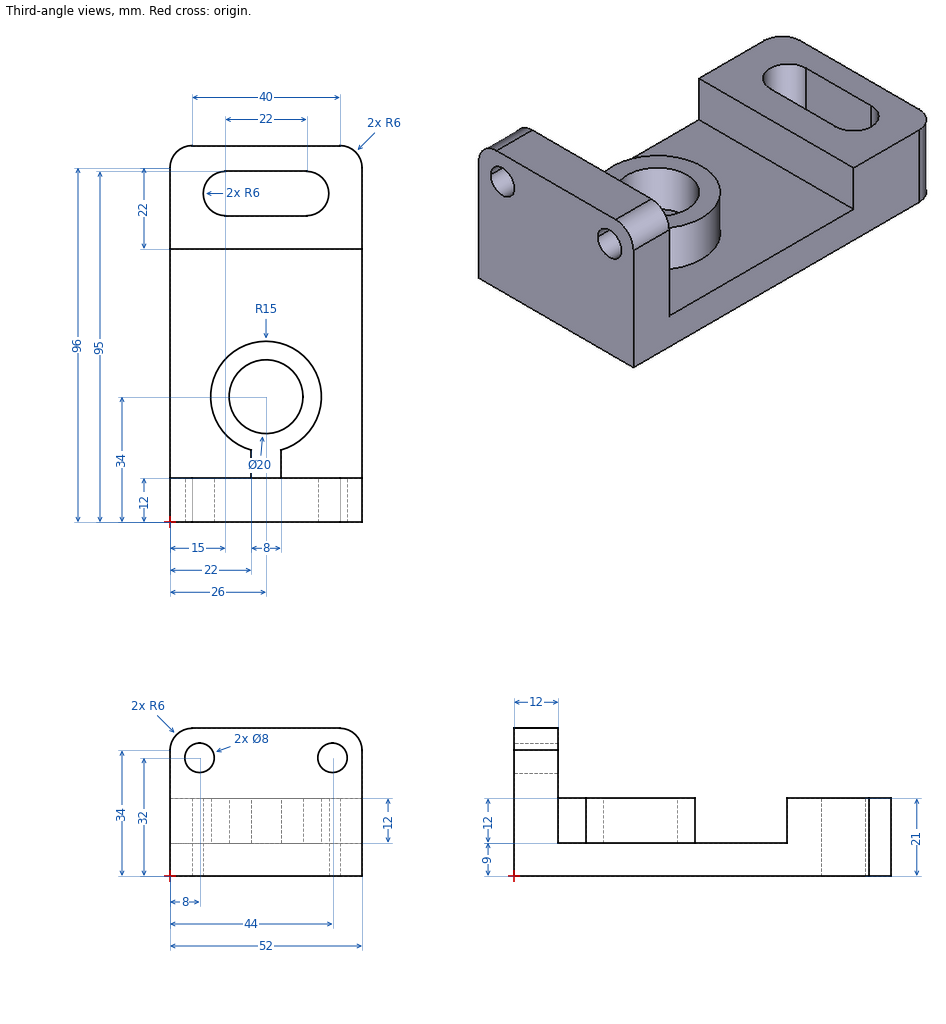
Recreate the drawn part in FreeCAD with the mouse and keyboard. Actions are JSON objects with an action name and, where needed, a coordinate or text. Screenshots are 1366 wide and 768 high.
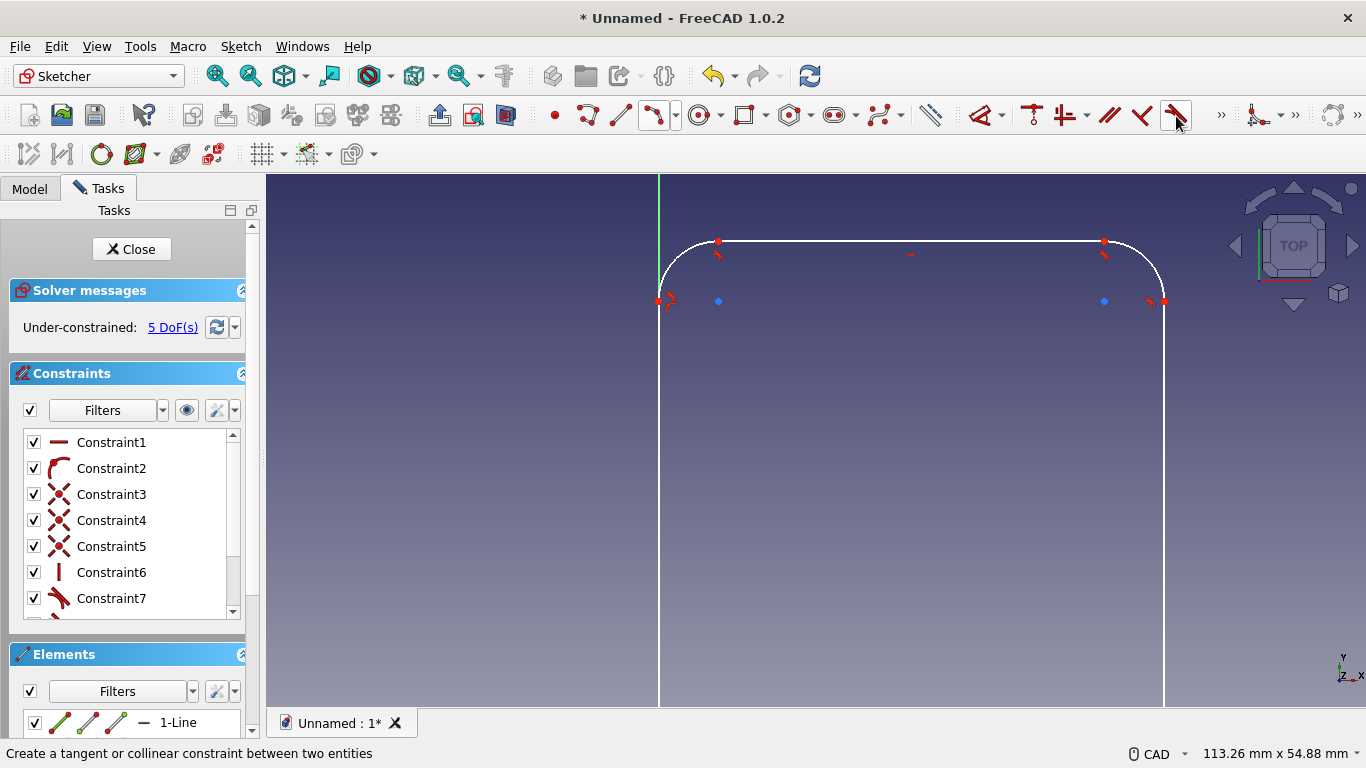
{"action": "scroll", "coordinate": [652, 270], "scroll_direction": "down", "scroll_amount": 5}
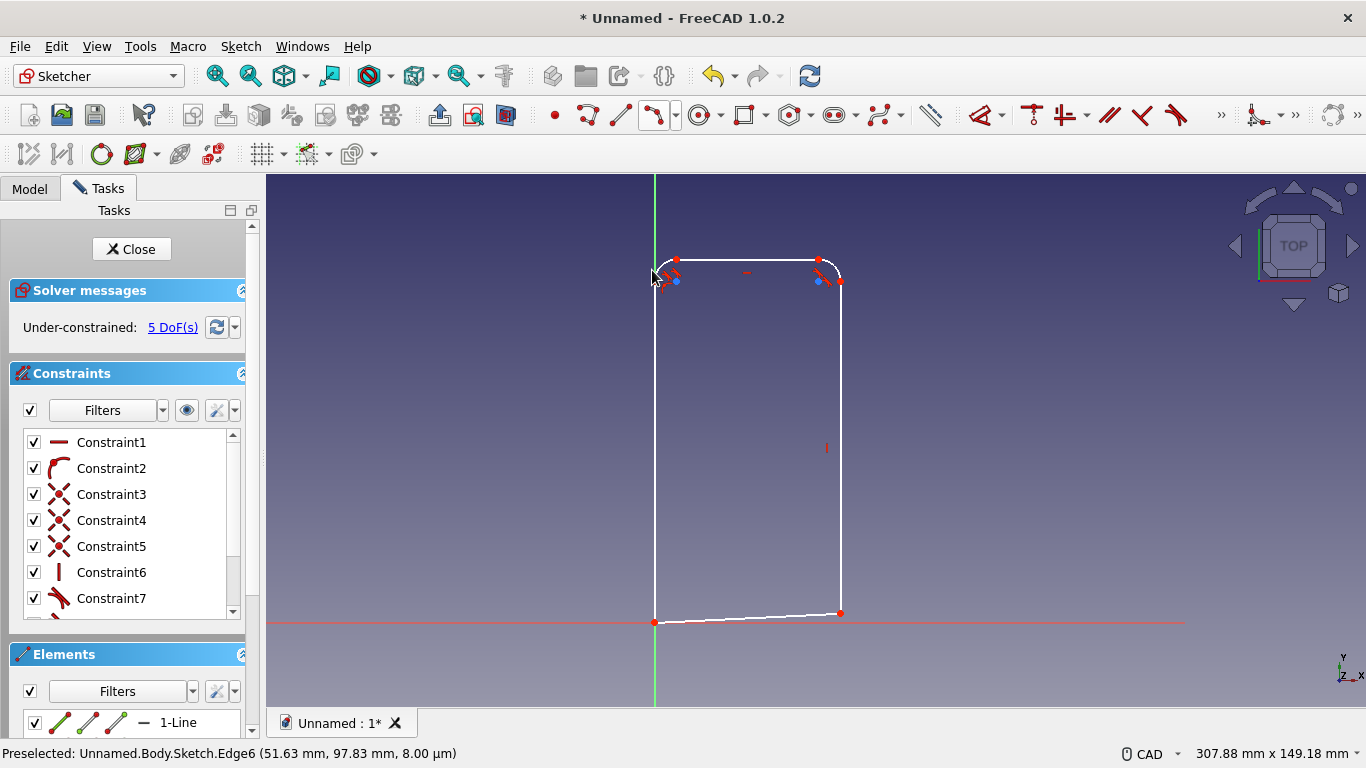
{"action": "scroll", "coordinate": [785, 617], "scroll_direction": "up", "scroll_amount": 4}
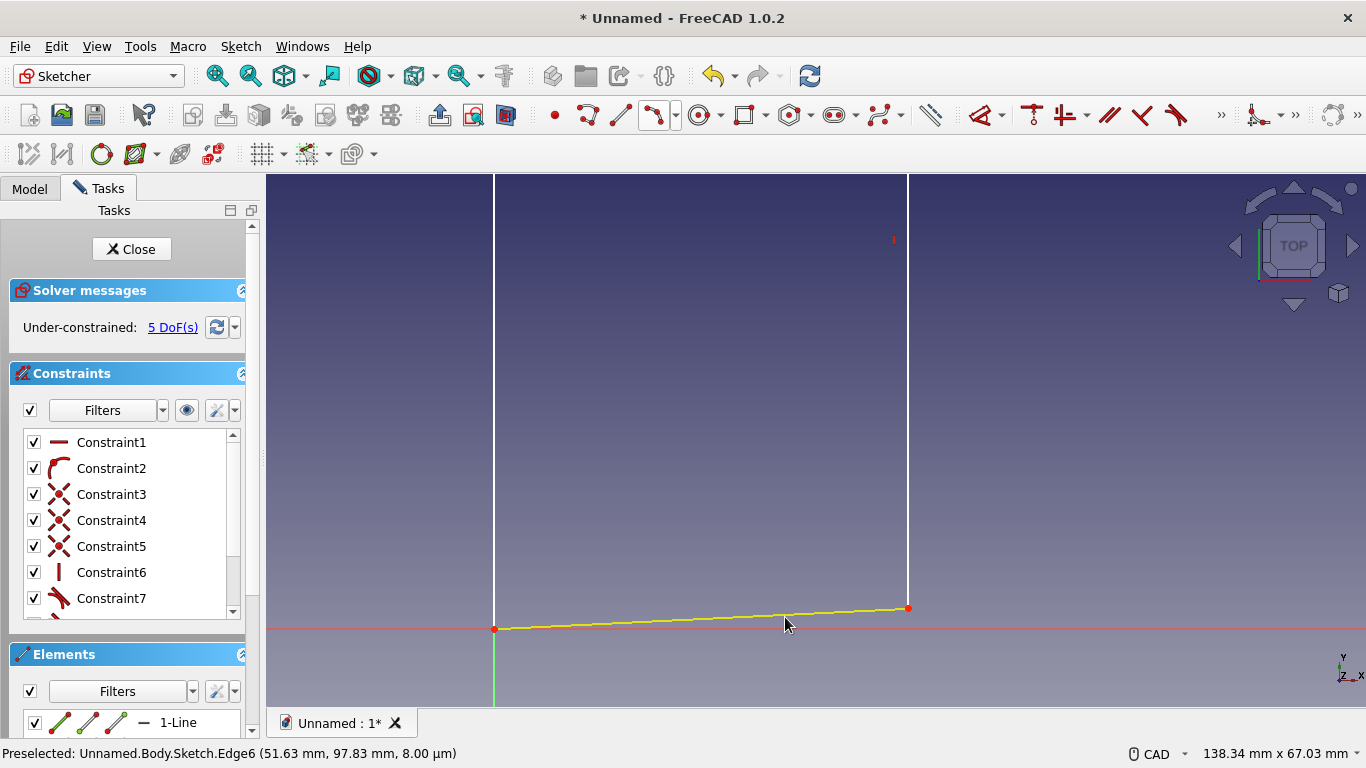
{"action": "left_click", "coordinate": [784, 615]}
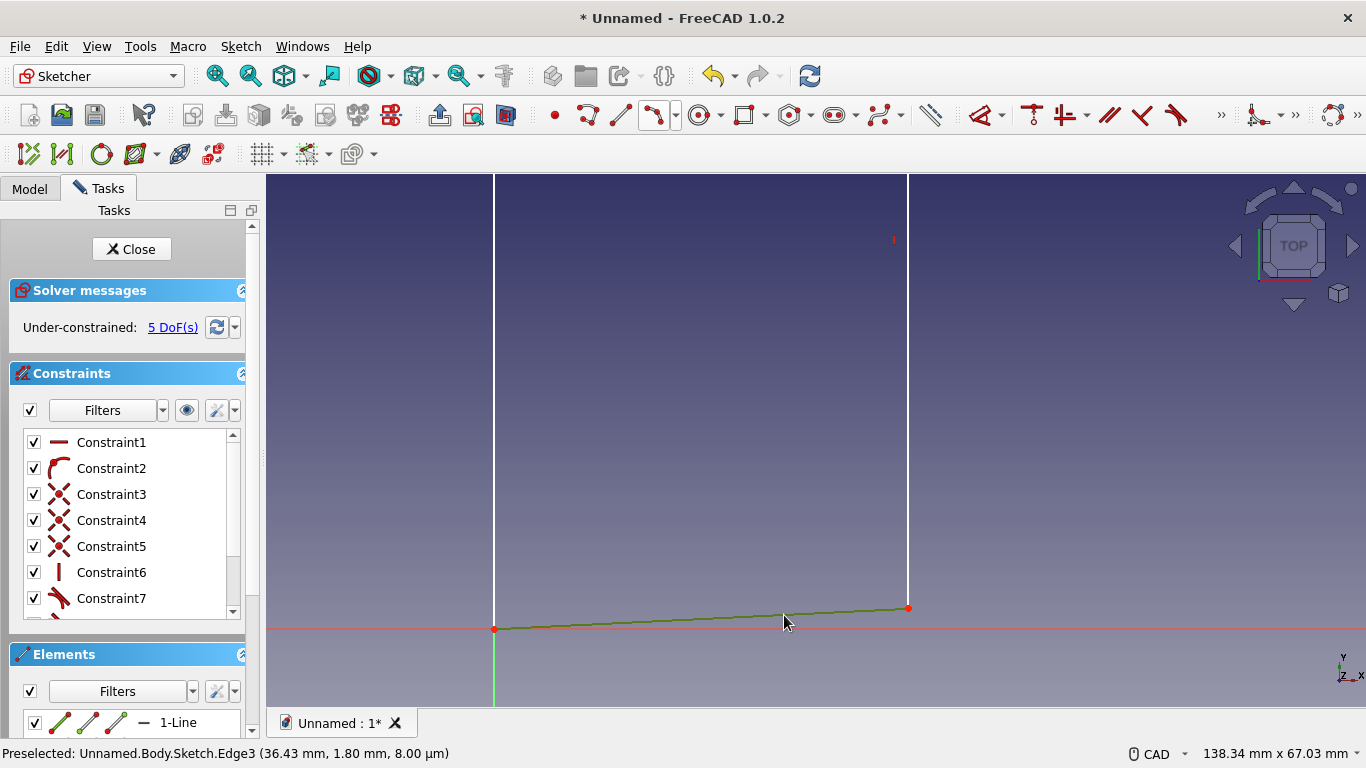
{"action": "key", "text": "h"}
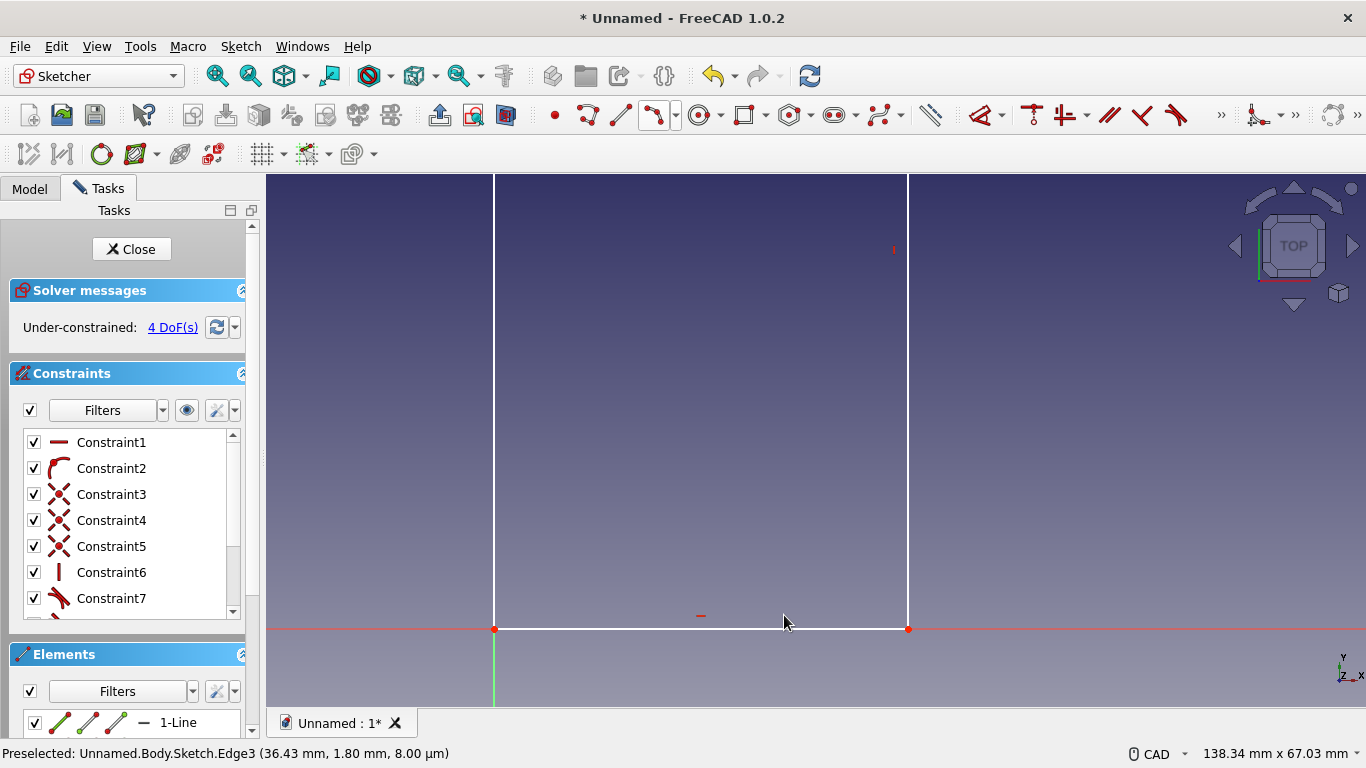
{"action": "scroll", "coordinate": [785, 617], "scroll_direction": "down", "scroll_amount": 4}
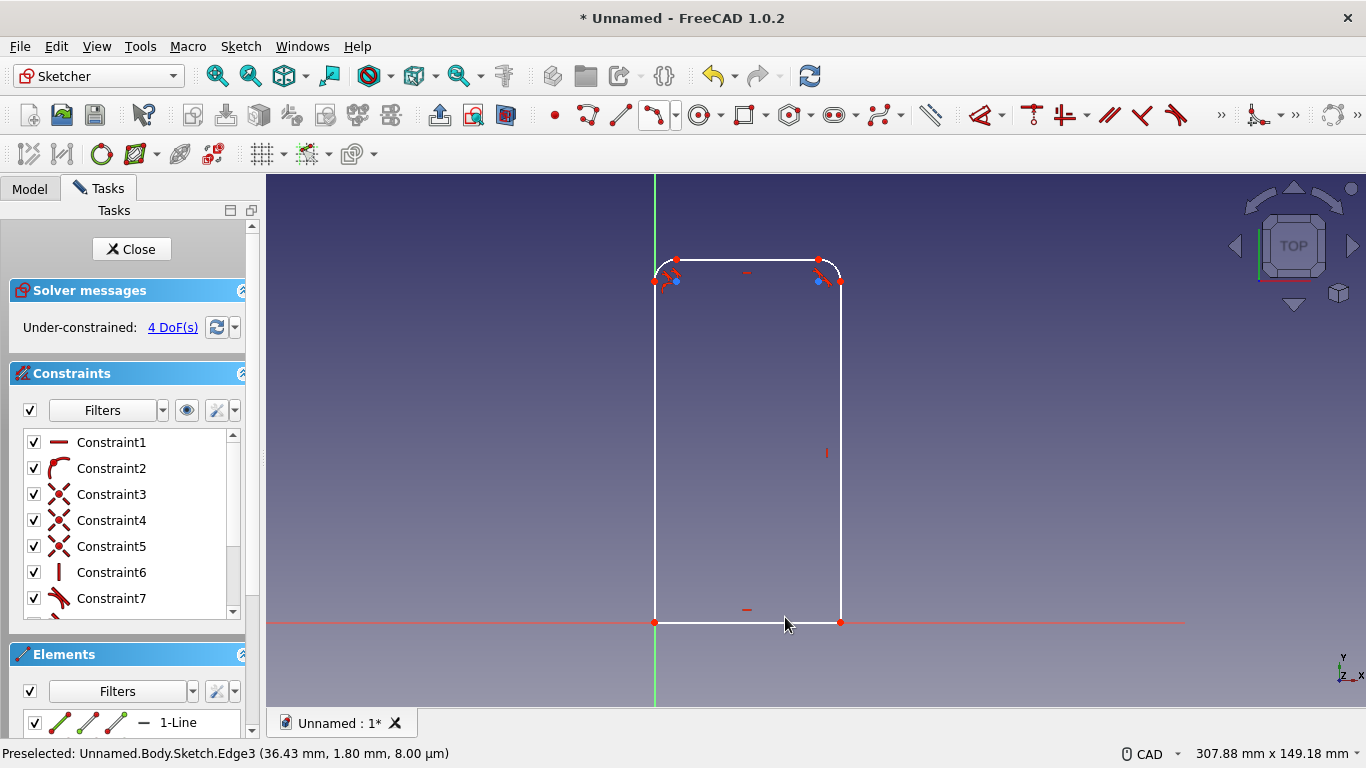
{"action": "scroll", "coordinate": [667, 262], "scroll_direction": "up", "scroll_amount": 2}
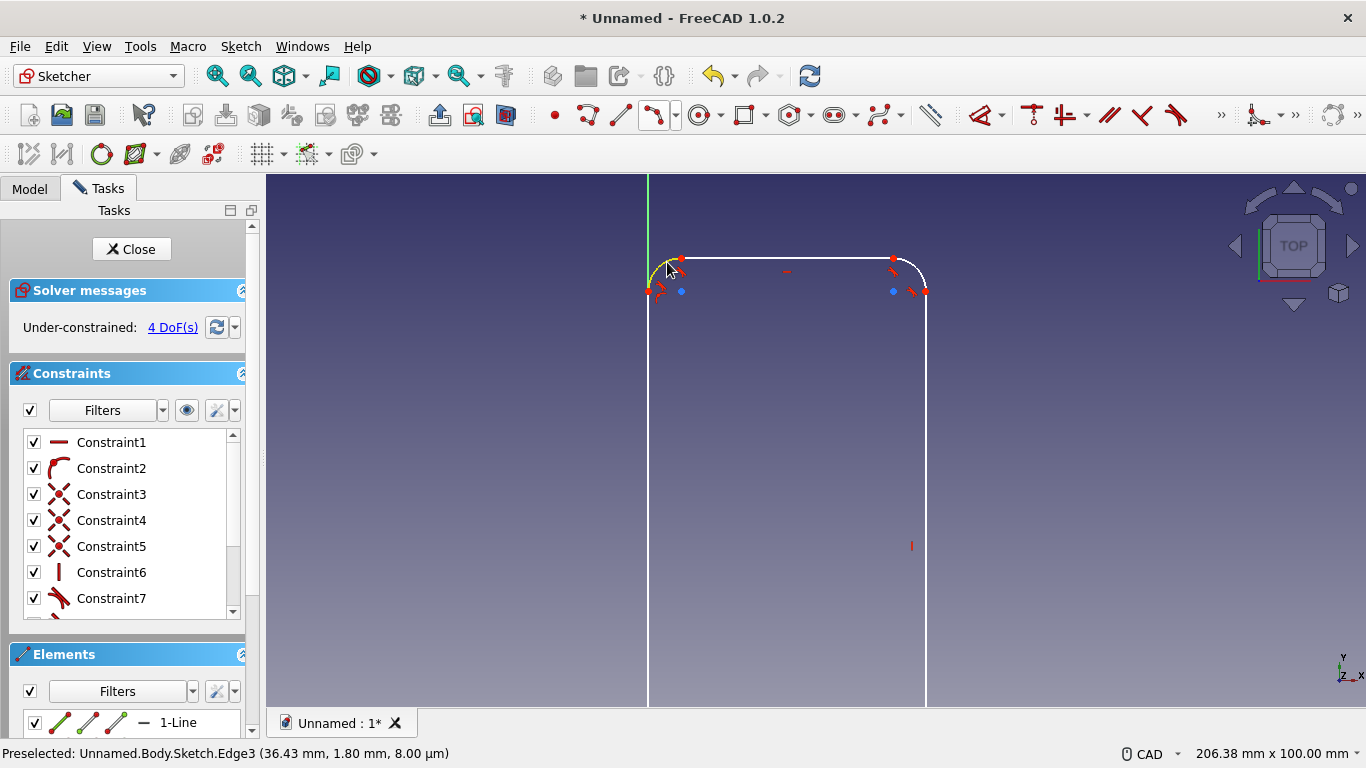
{"action": "left_click", "coordinate": [666, 262]}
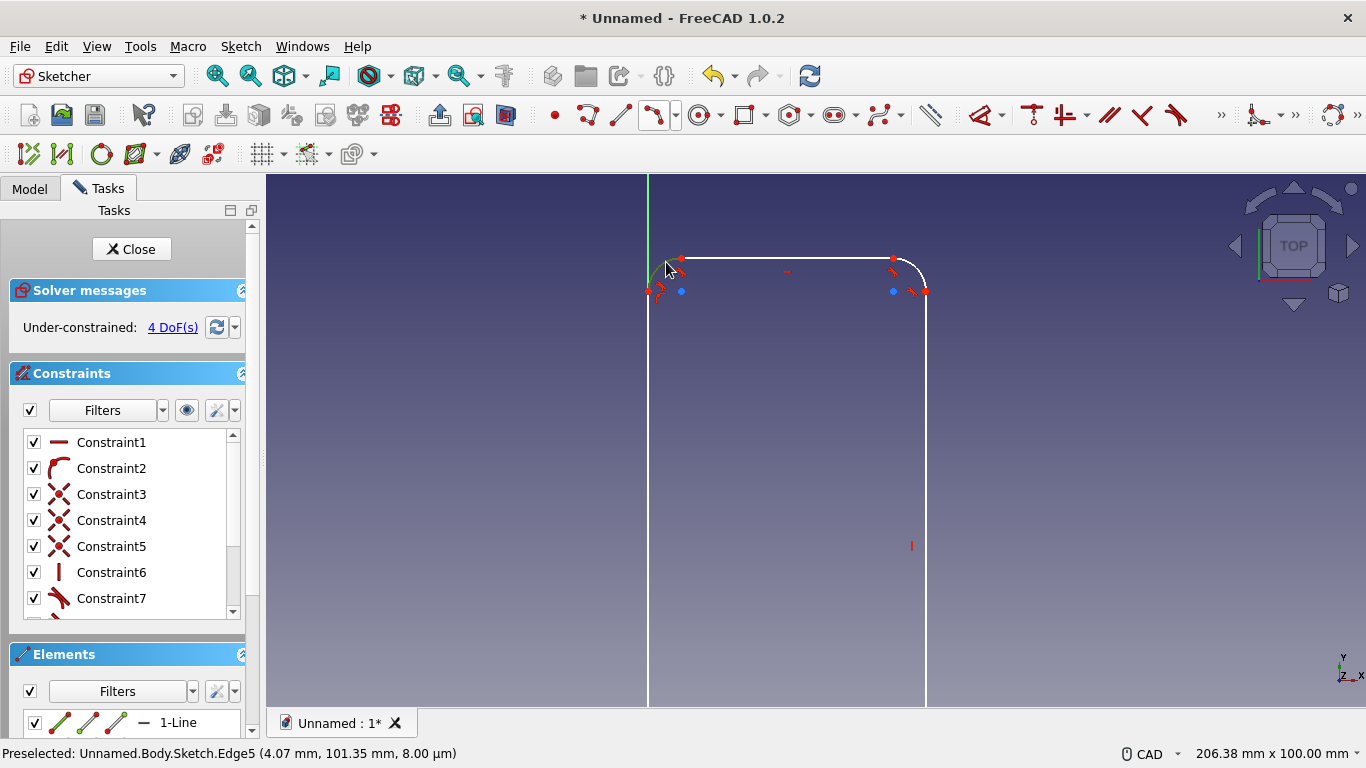
{"action": "left_click", "coordinate": [922, 276]}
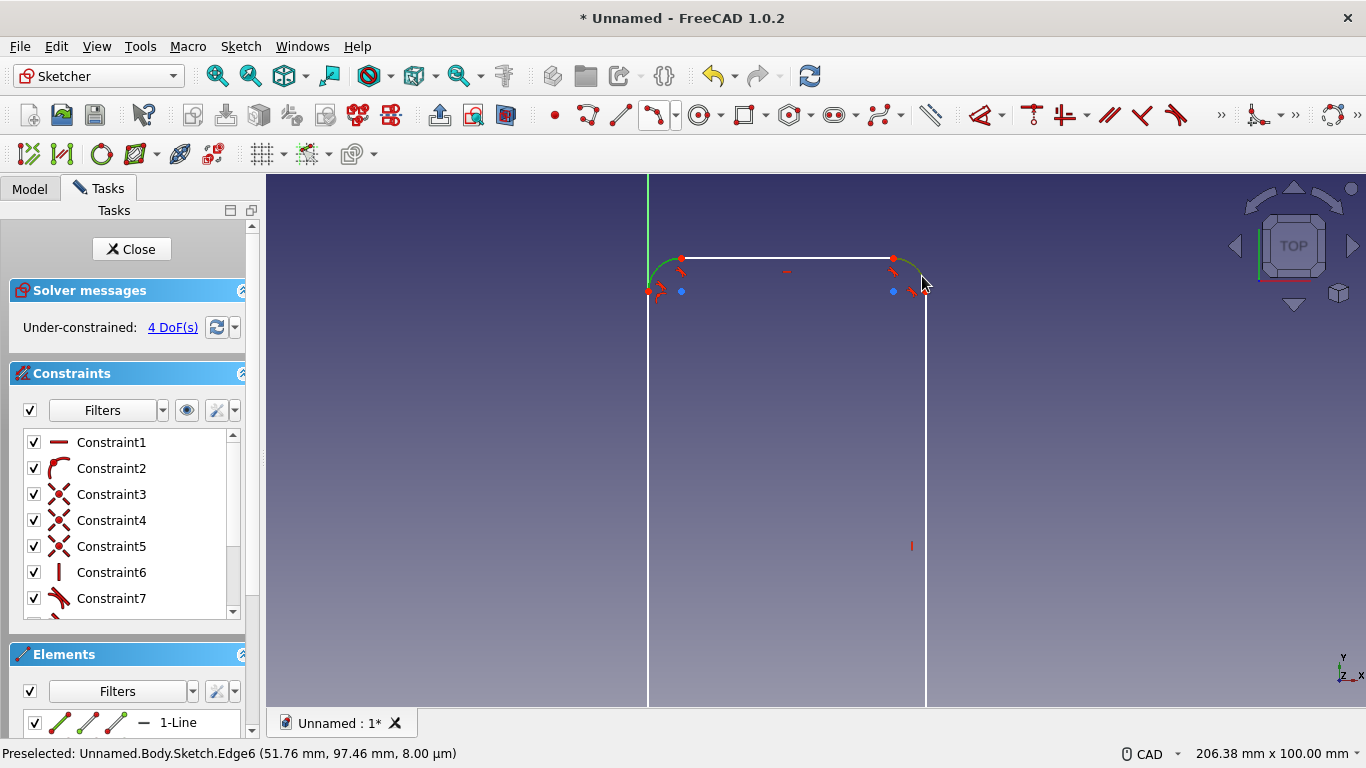
{"action": "key", "text": "e"}